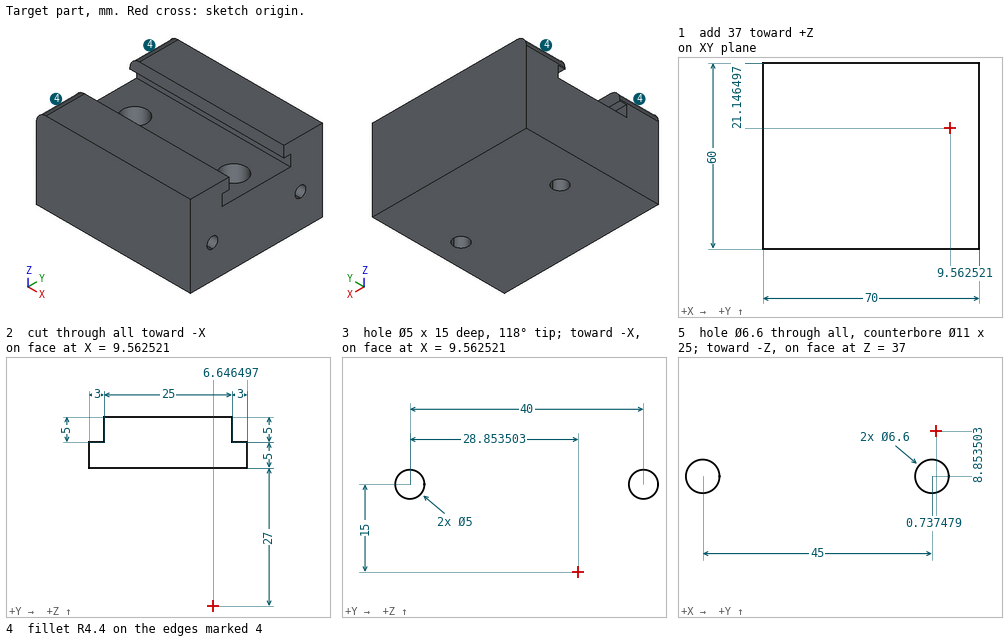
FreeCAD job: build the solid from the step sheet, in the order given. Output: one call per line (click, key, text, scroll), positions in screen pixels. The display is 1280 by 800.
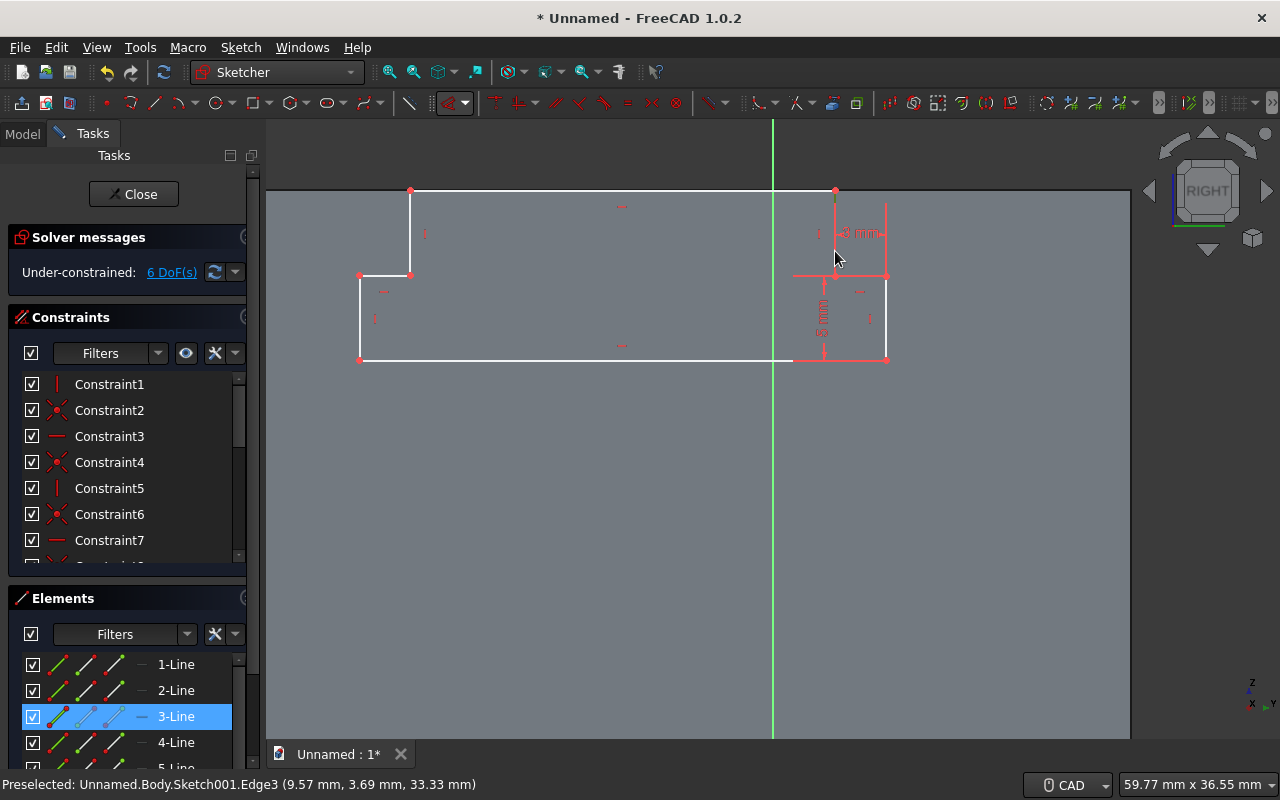
click(468, 104)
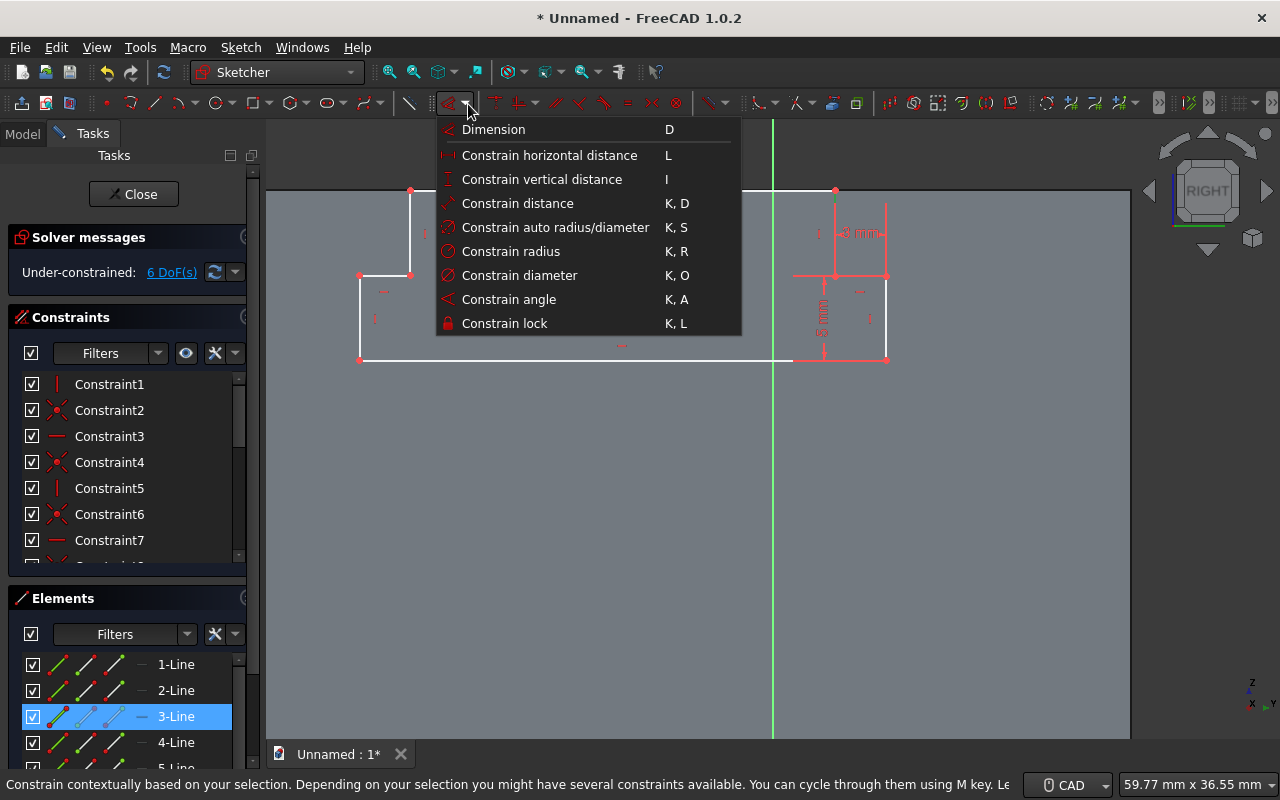
click(589, 179)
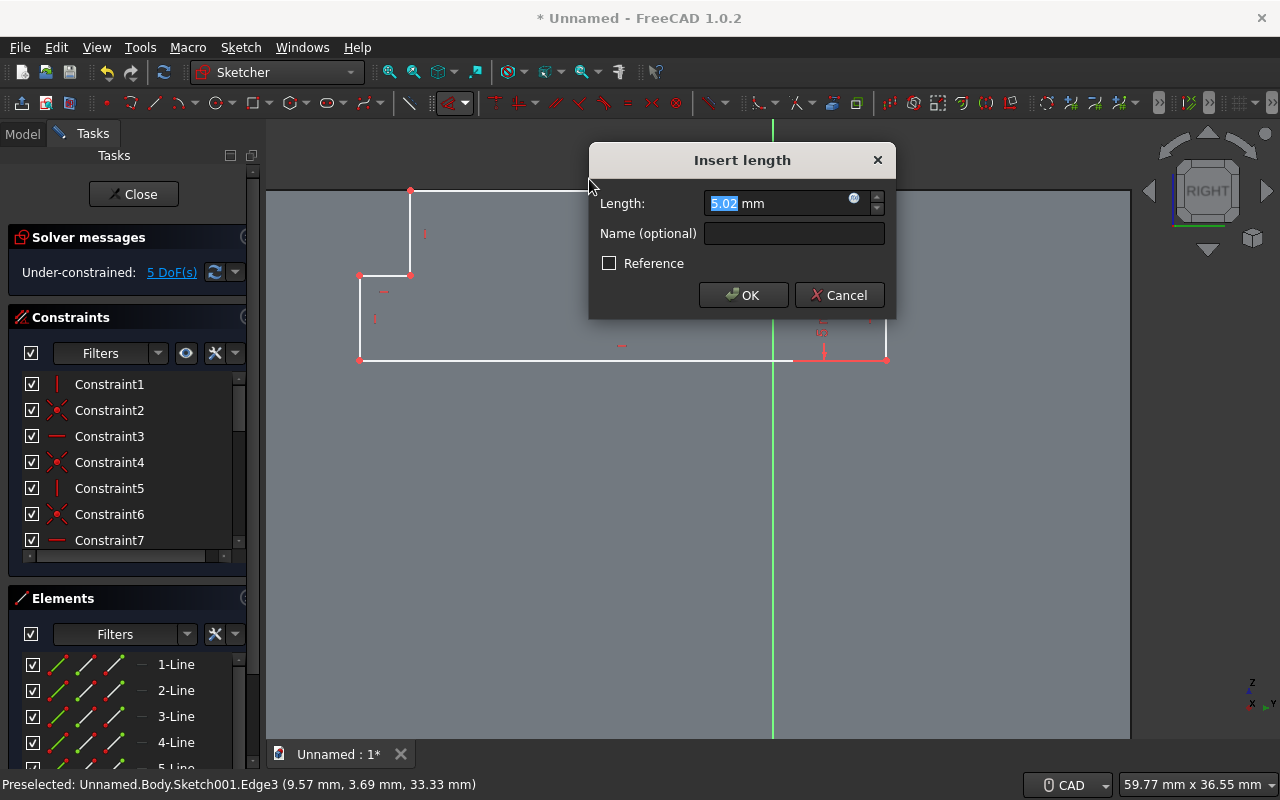
text(5)
key(Return)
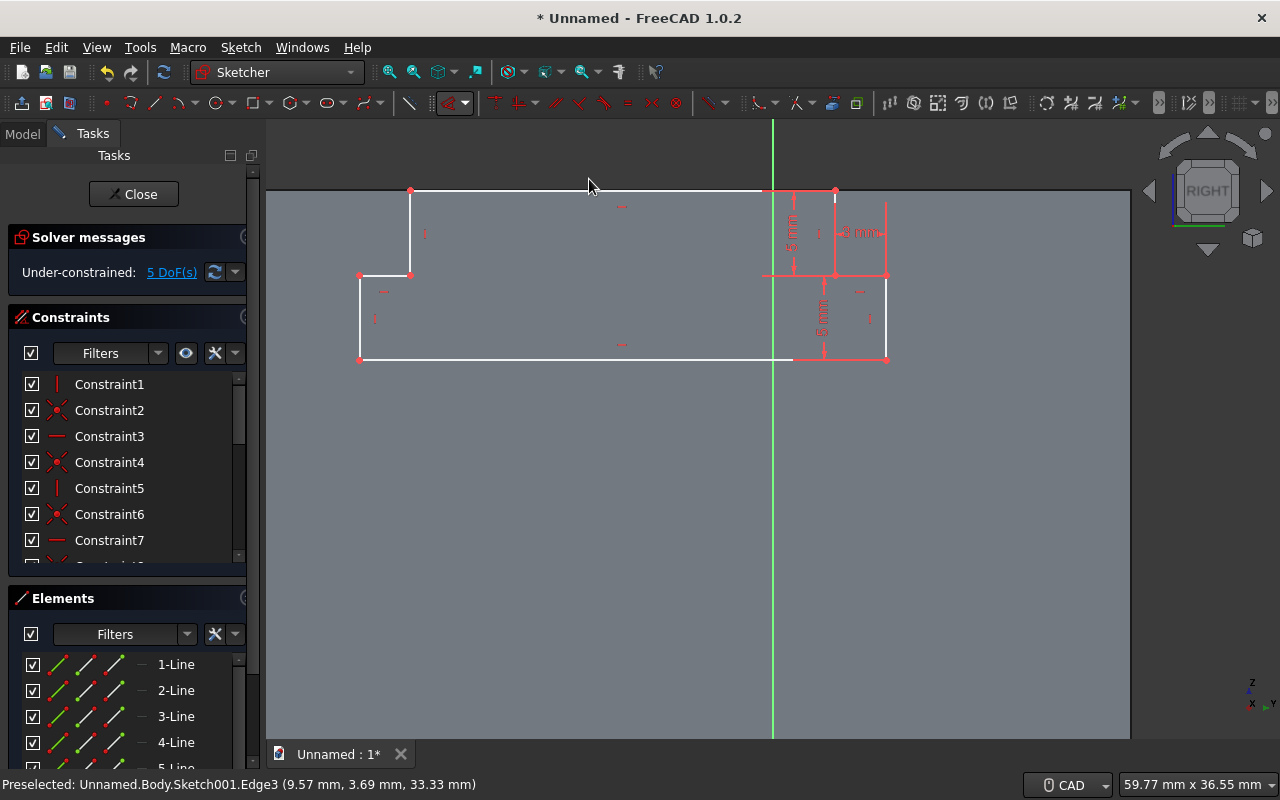
click(410, 216)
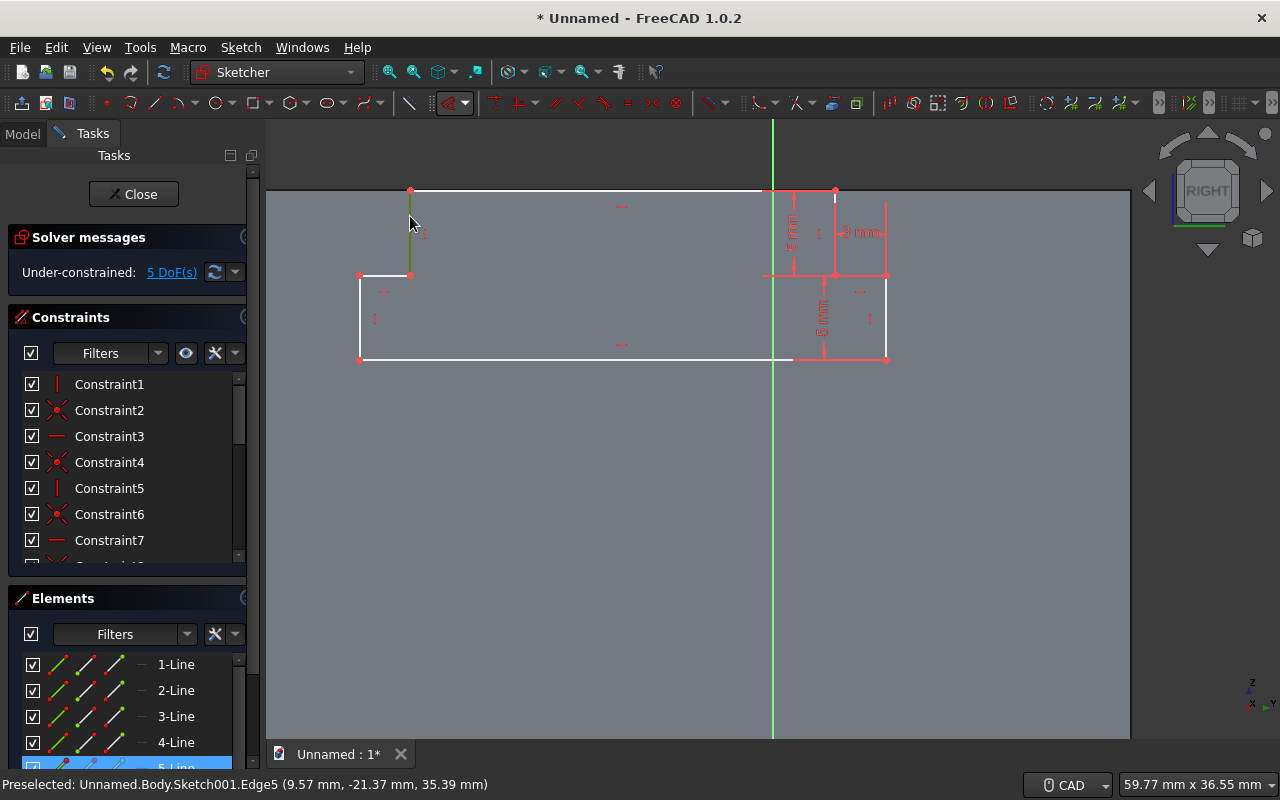
click(468, 104)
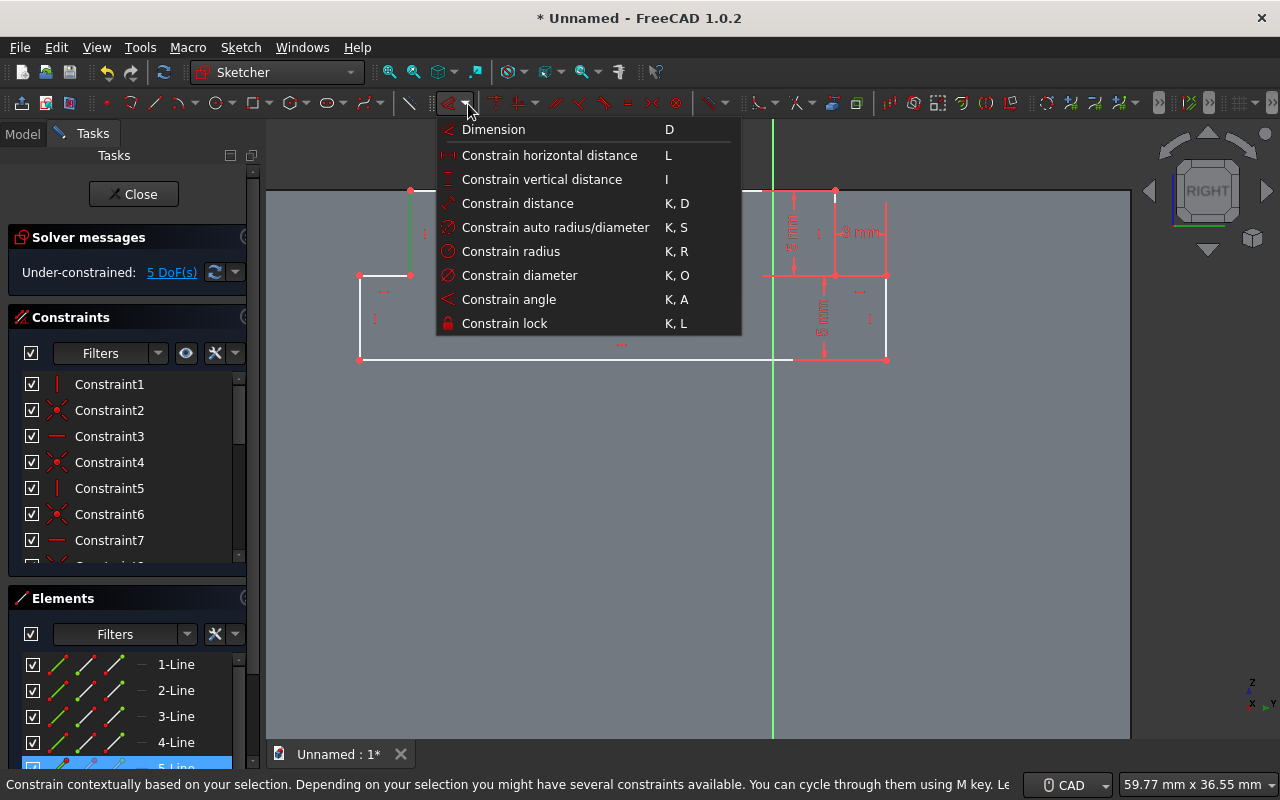
click(589, 179)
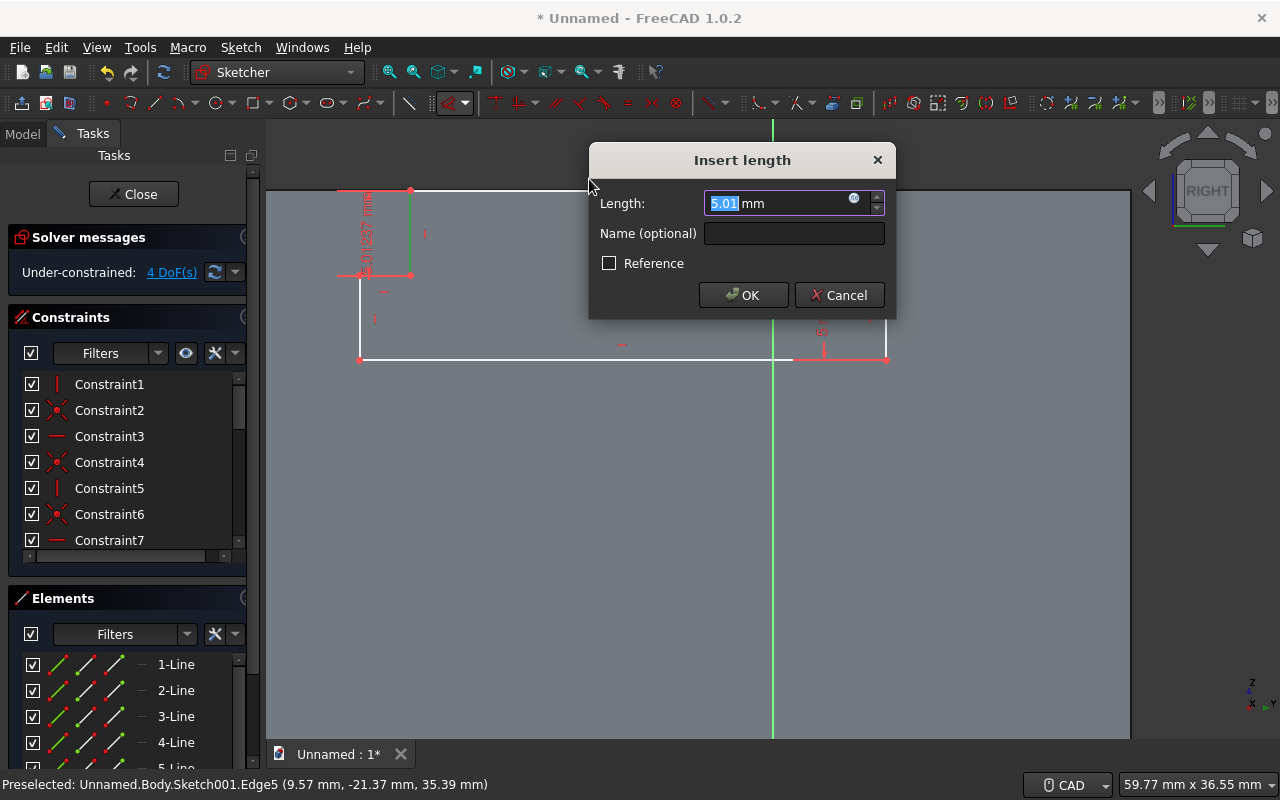
text(5)
key(Return)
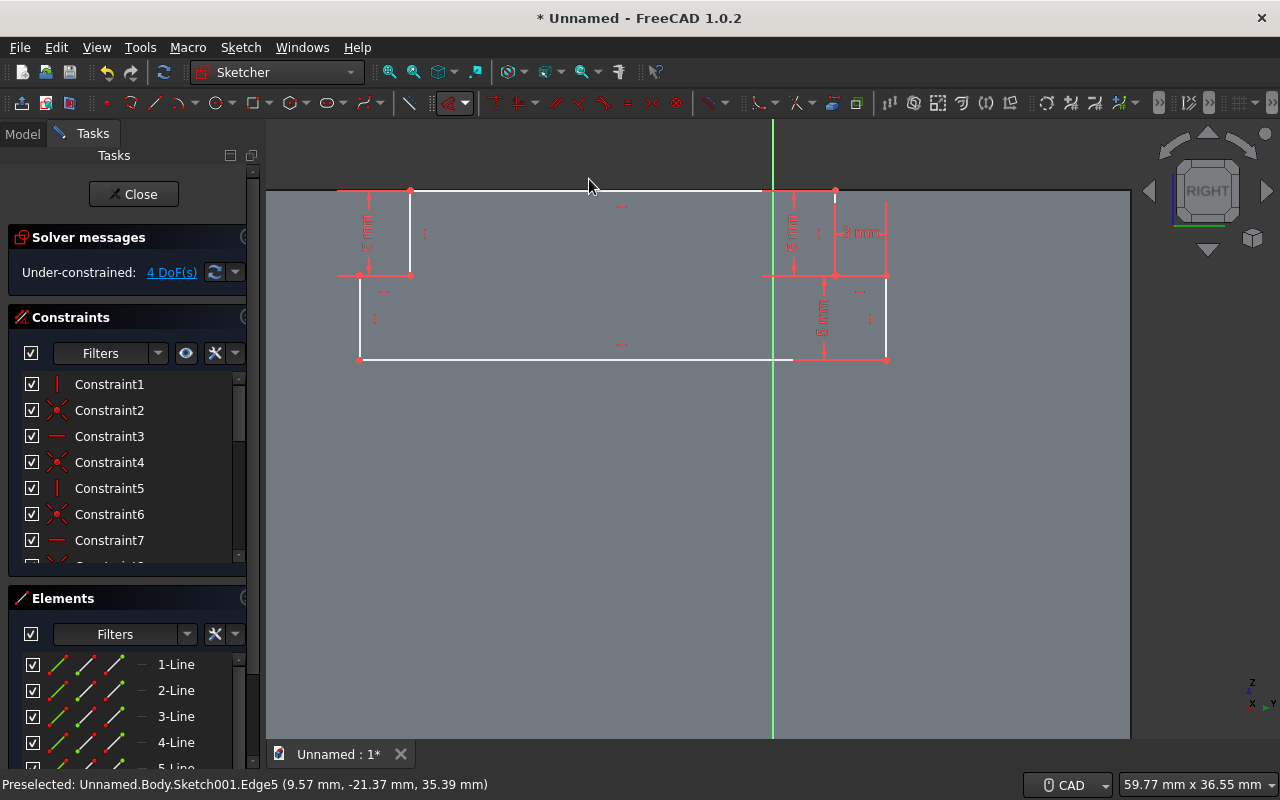
click(395, 276)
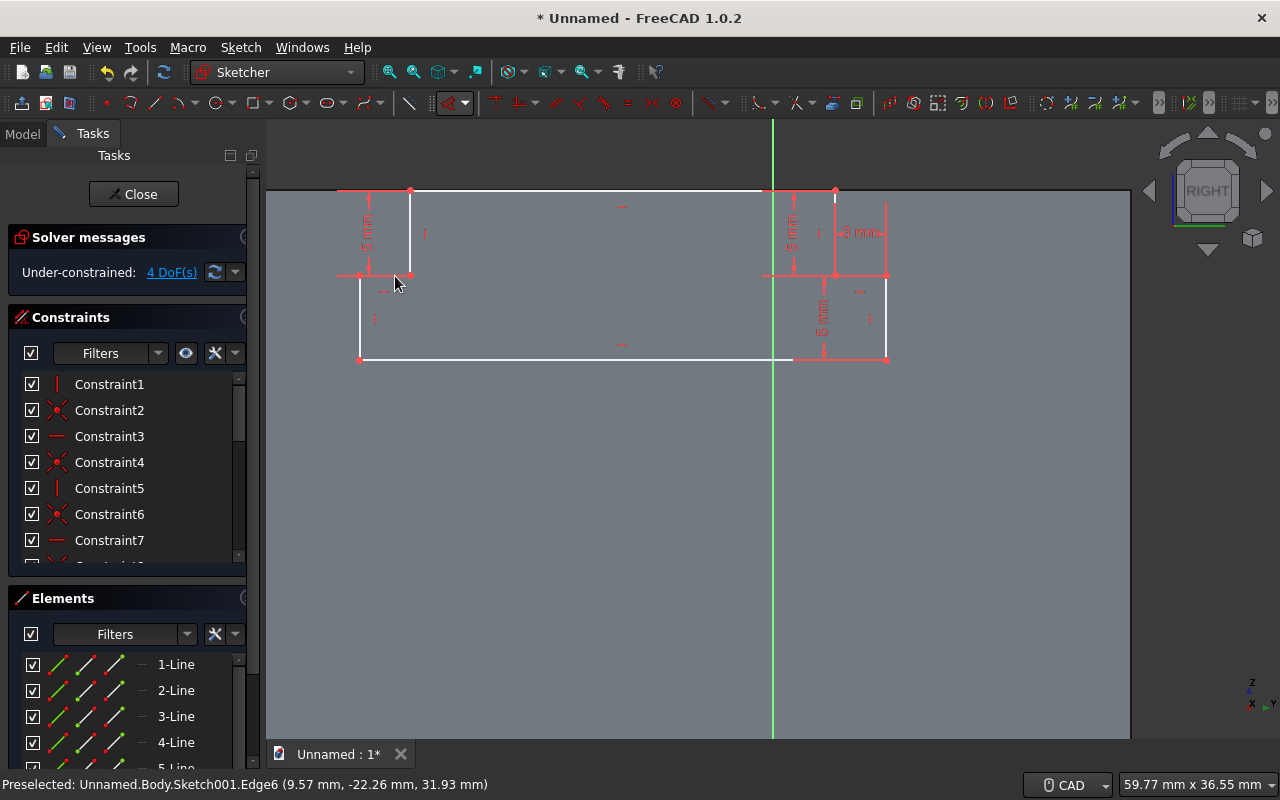
click(468, 104)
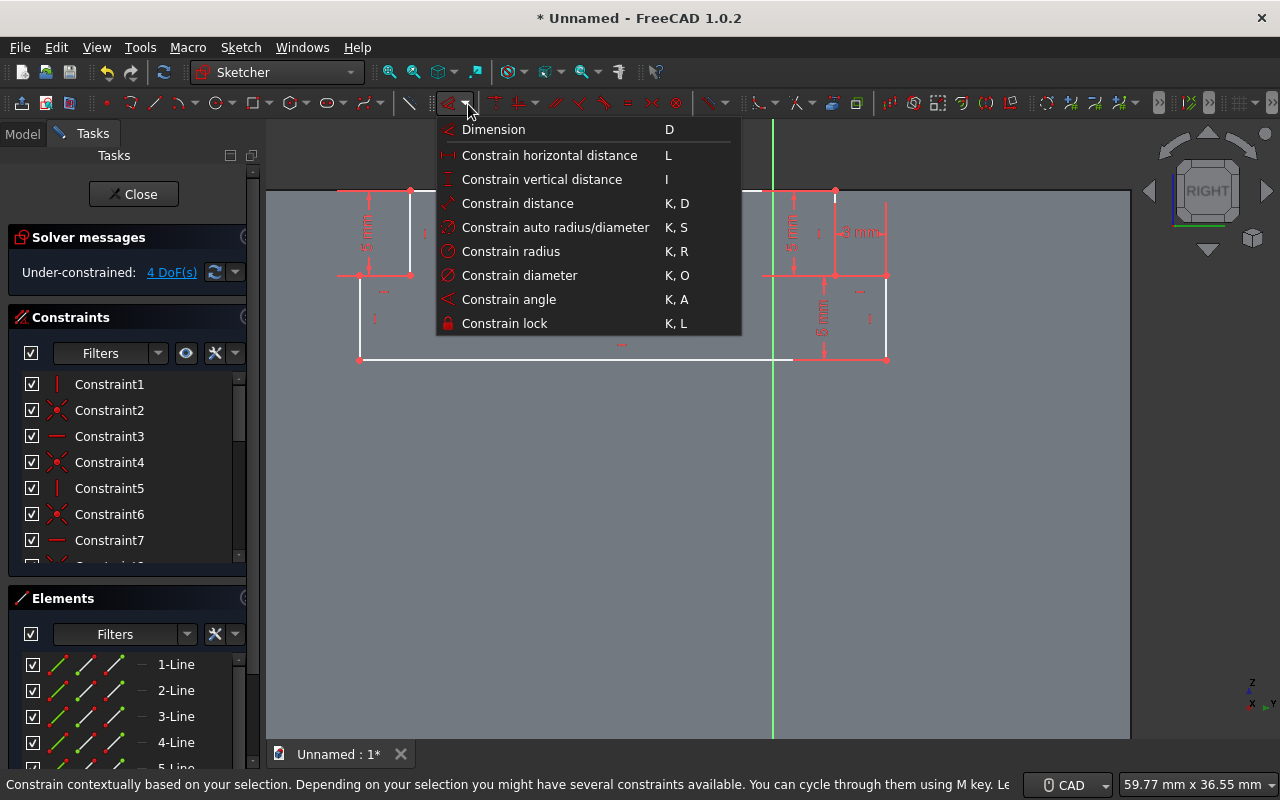
click(589, 155)